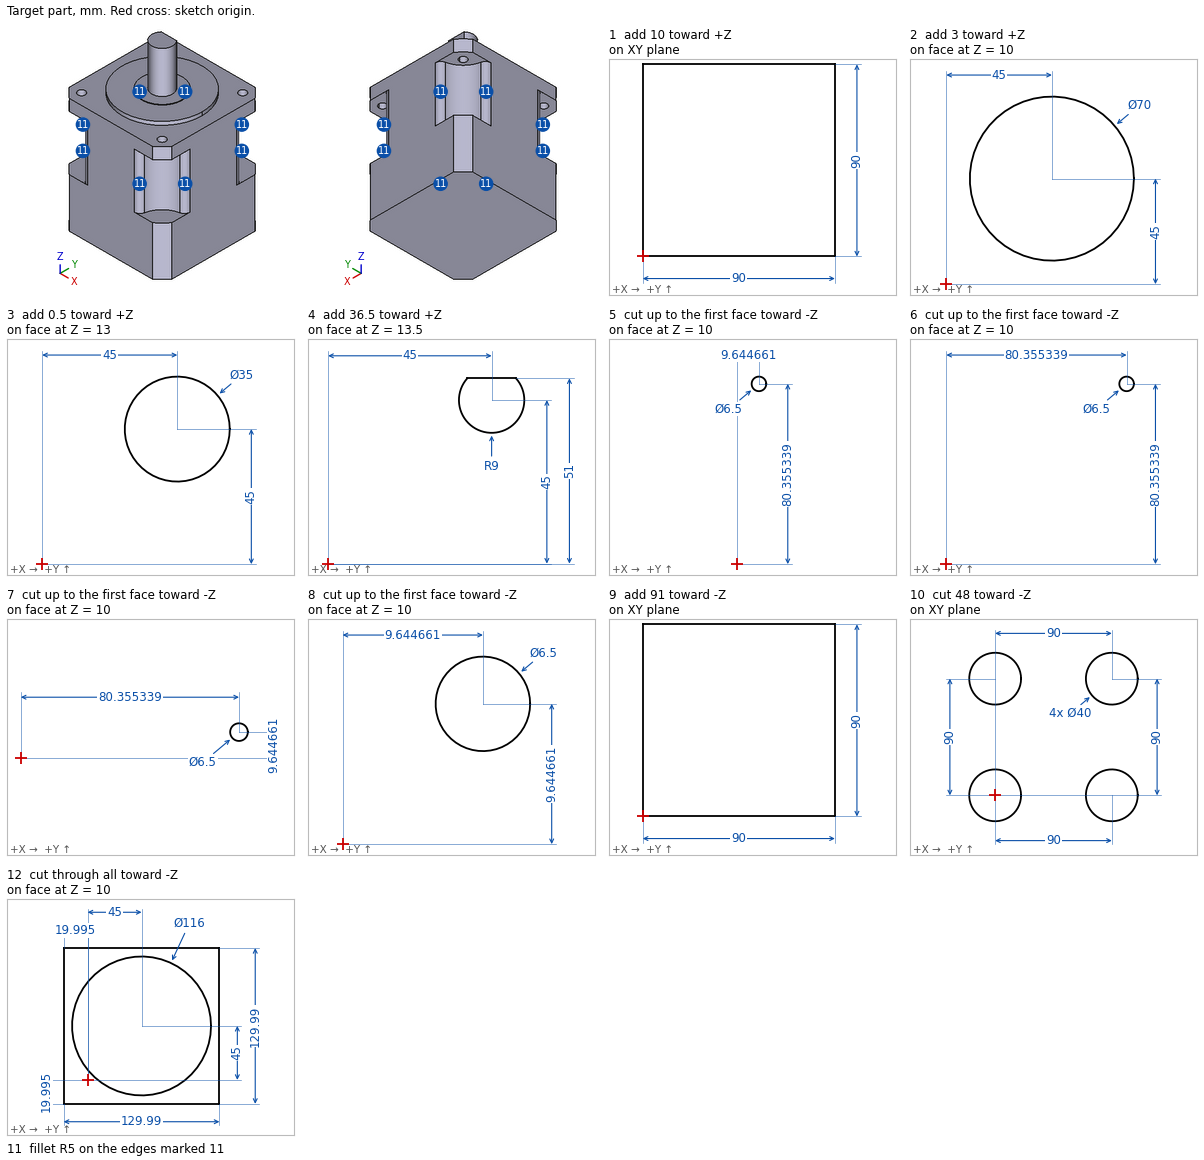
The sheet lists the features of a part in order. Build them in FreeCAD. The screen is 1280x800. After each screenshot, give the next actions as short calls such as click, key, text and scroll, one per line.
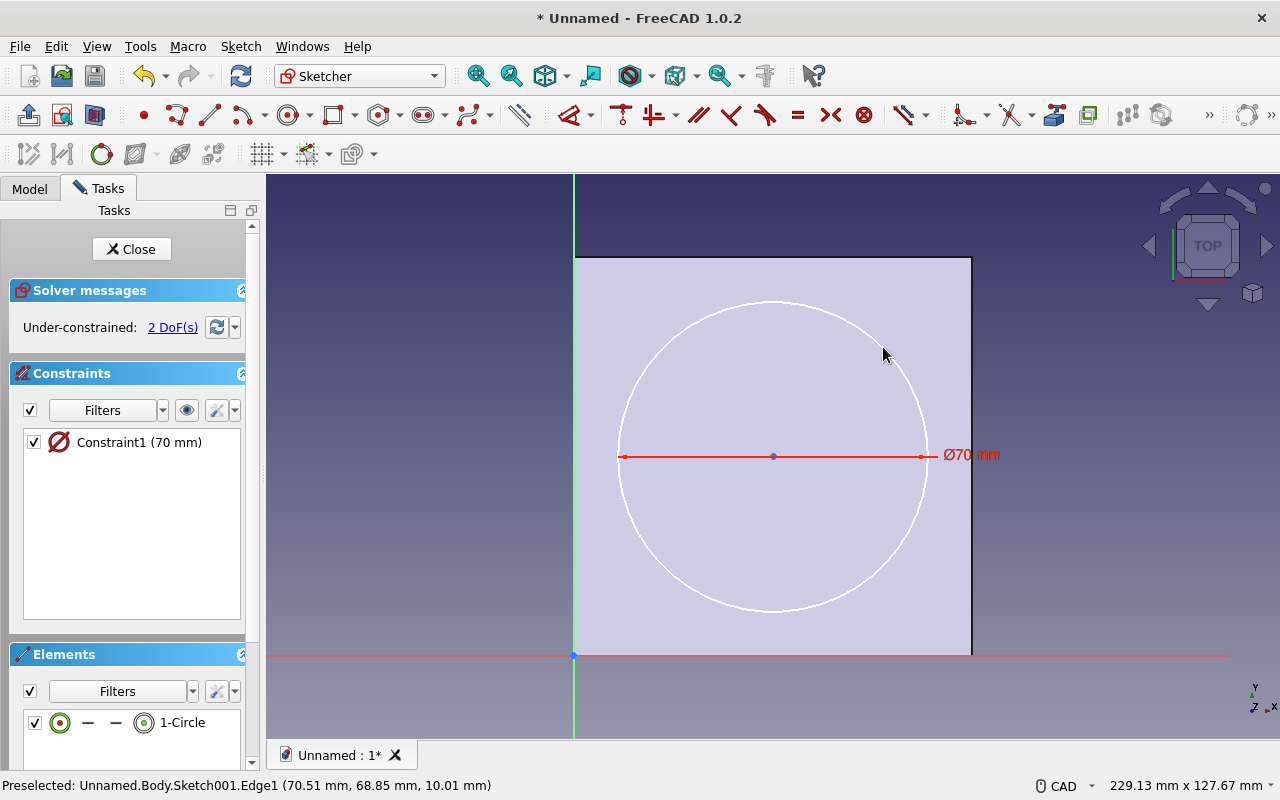
click(773, 457)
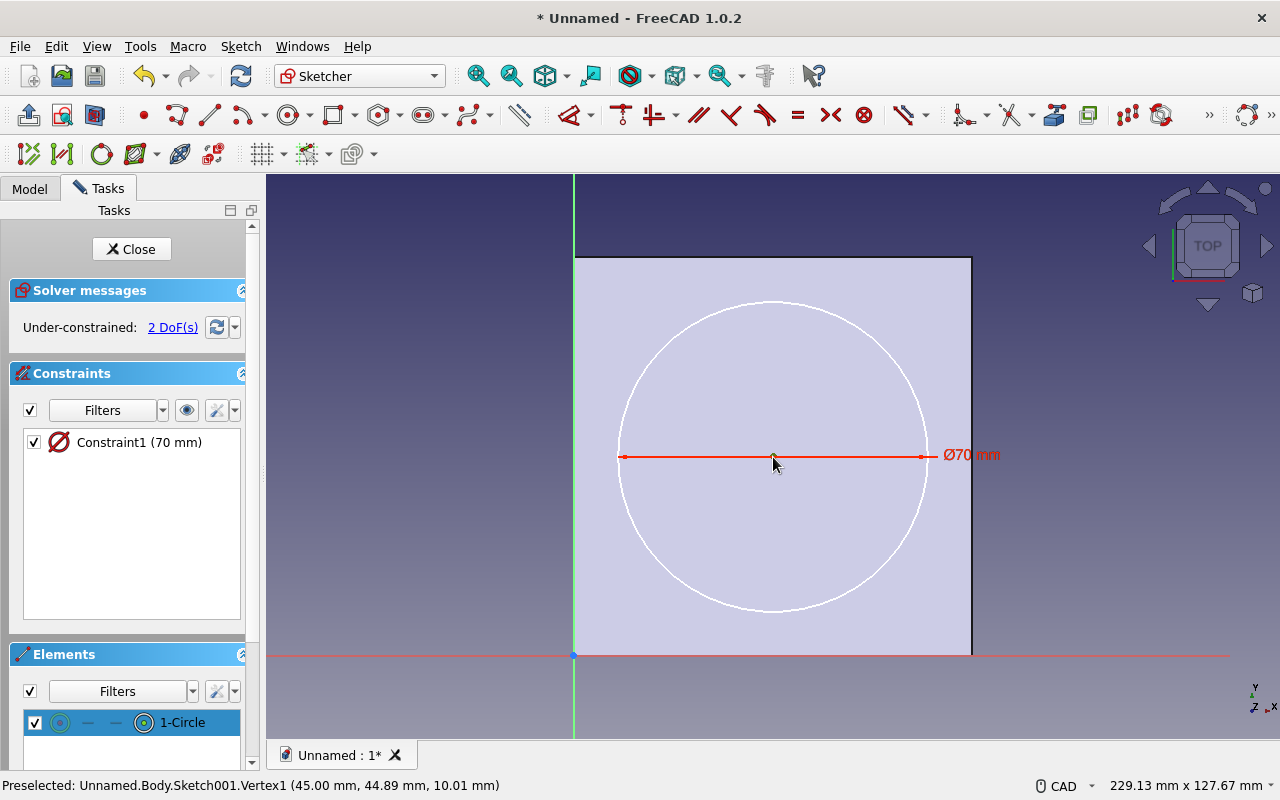
key(l)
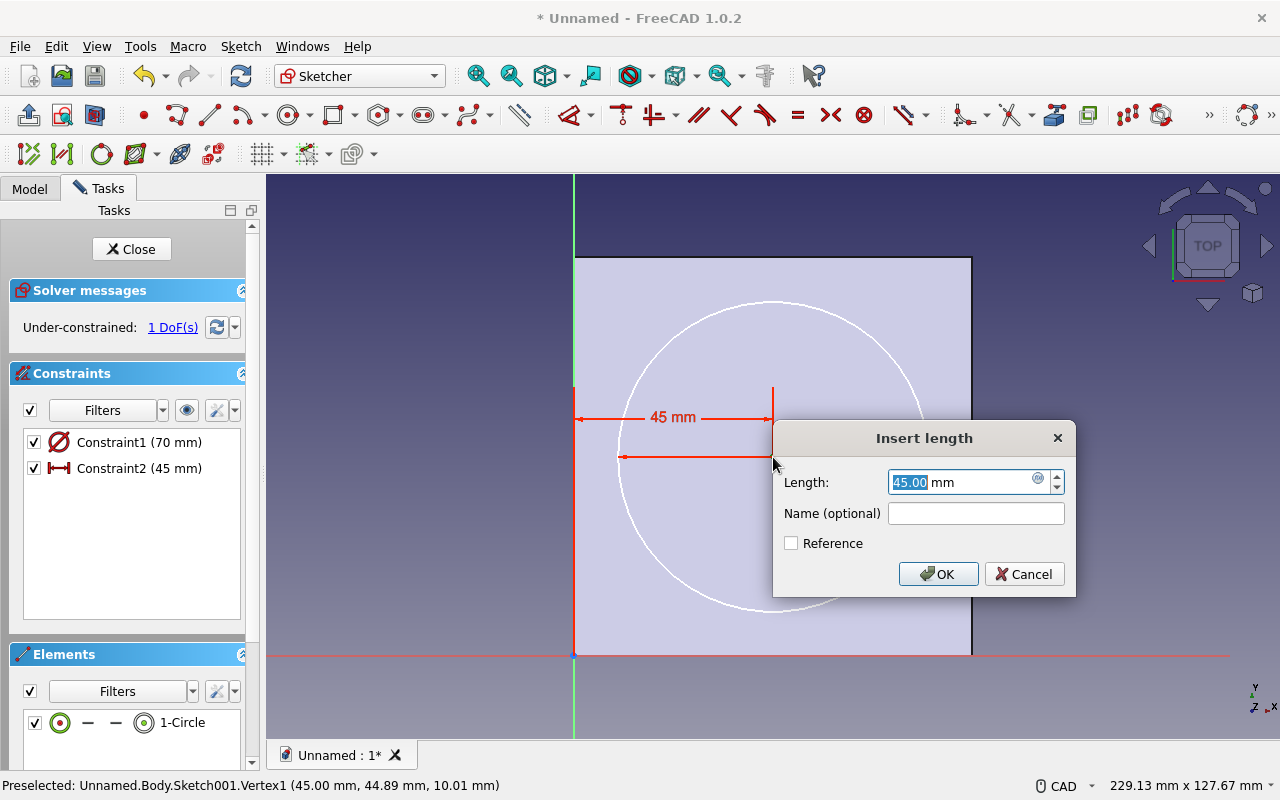
text(45)
key(Return)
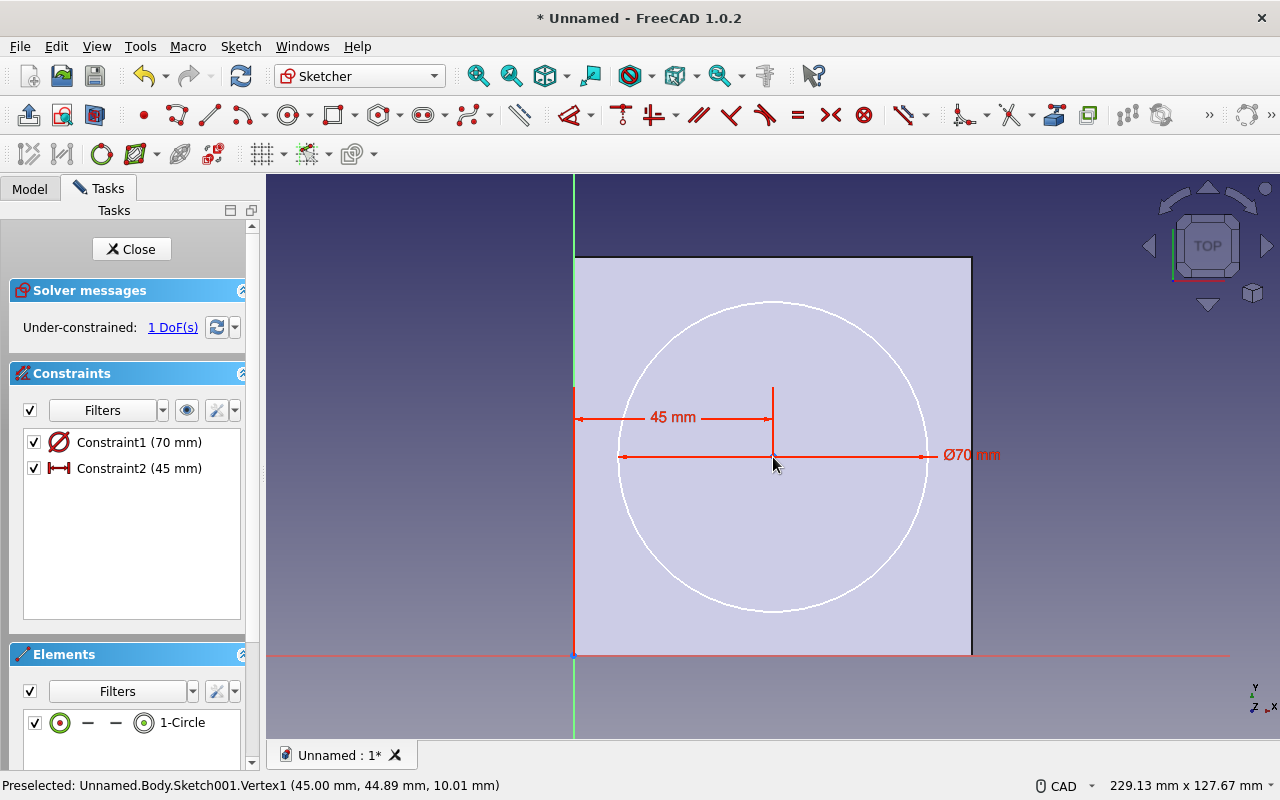
click(773, 457)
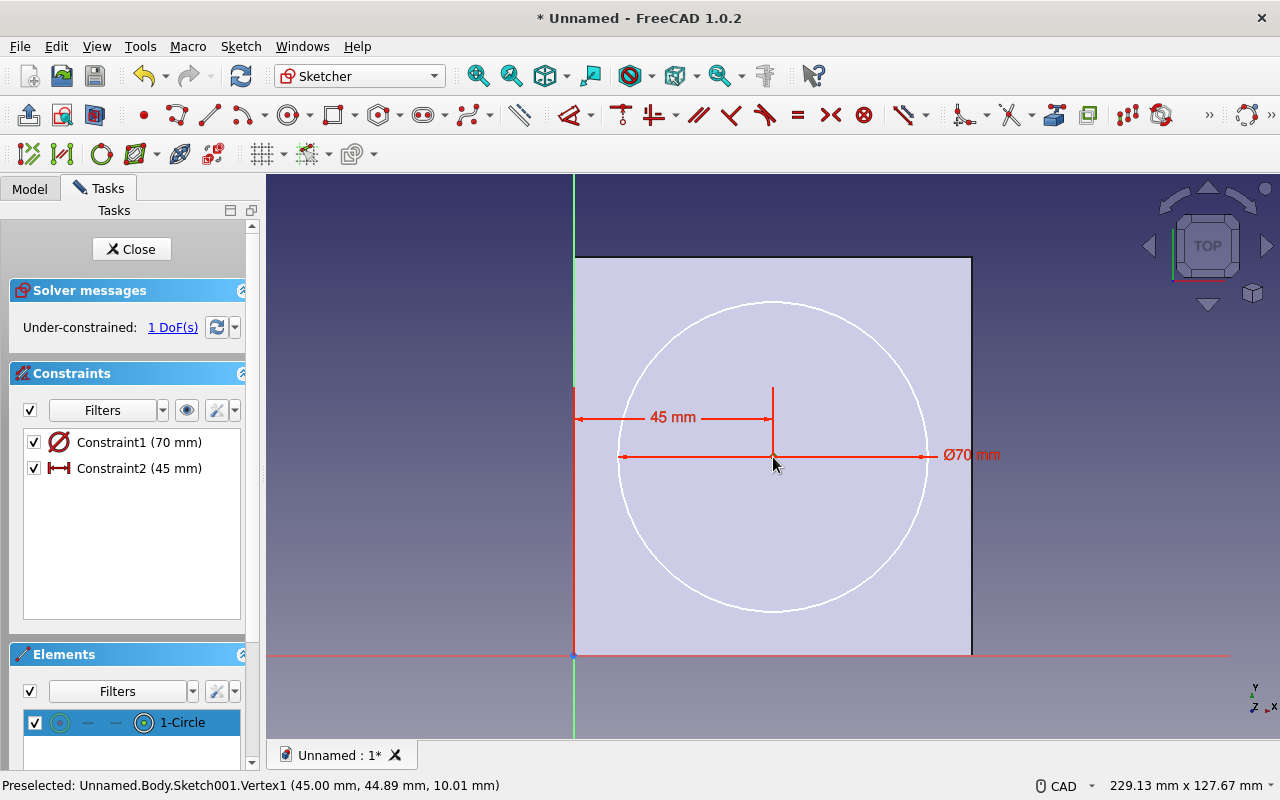
key(i)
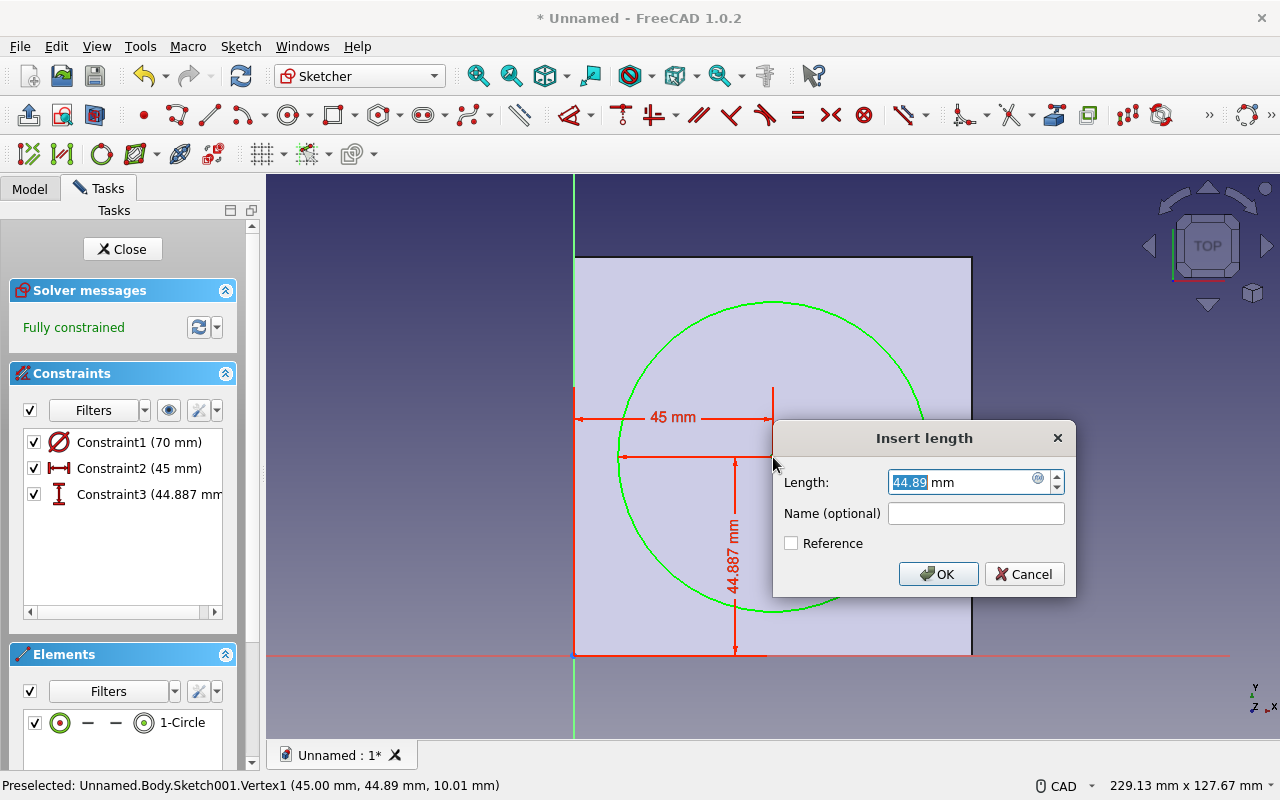
text(45)
key(Return)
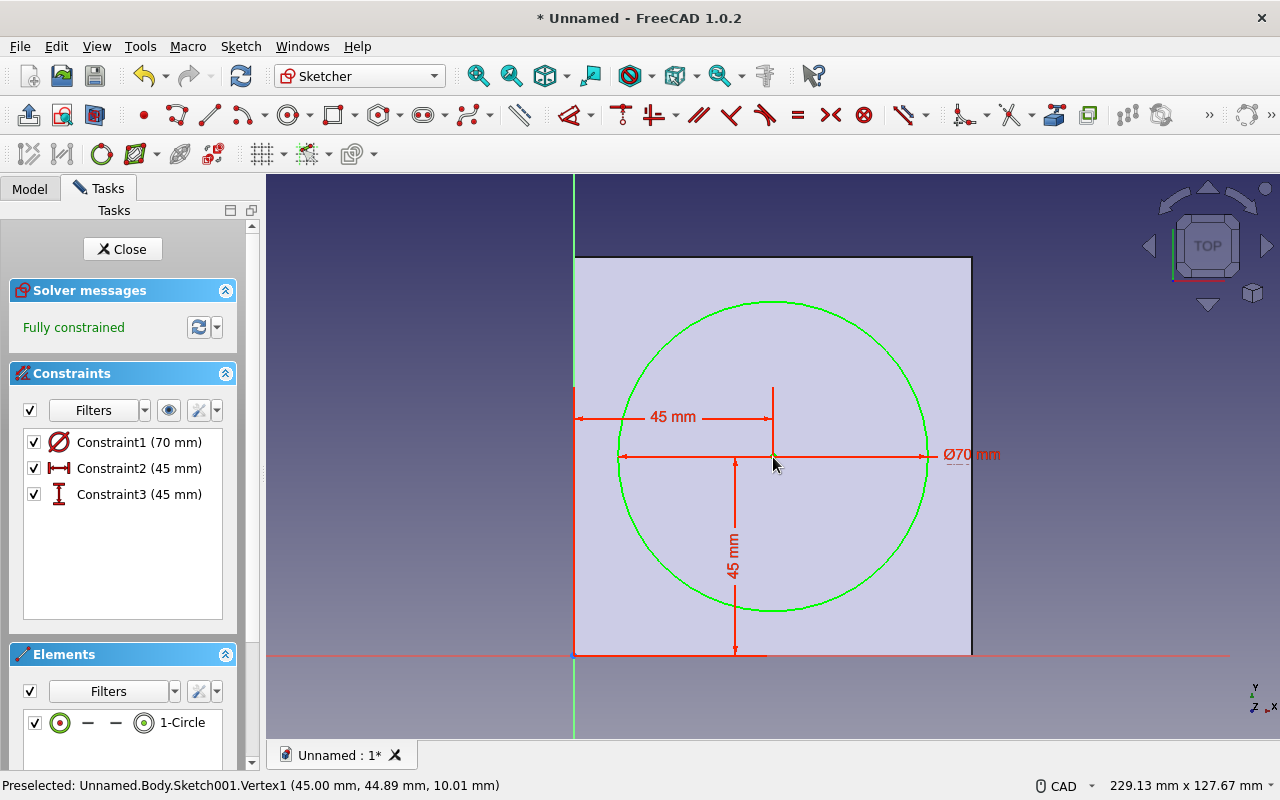
click(123, 249)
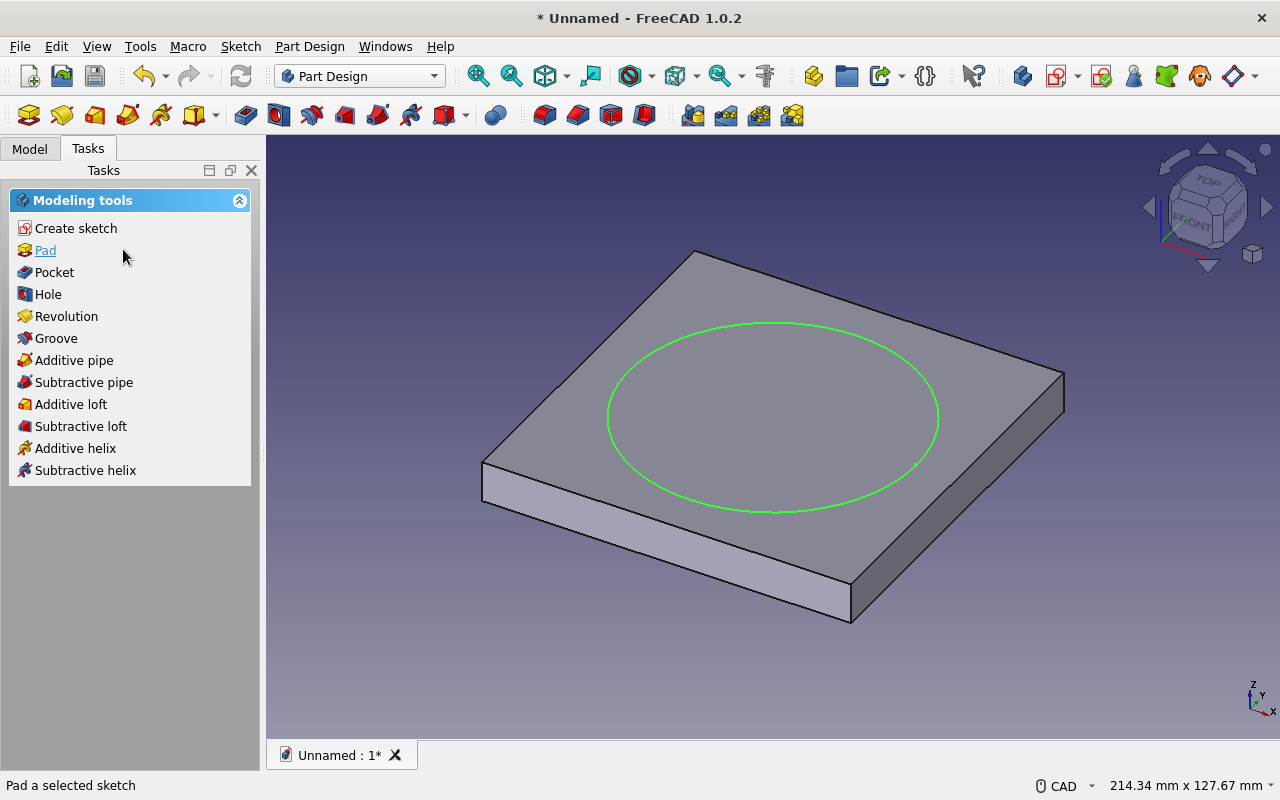
click(29, 116)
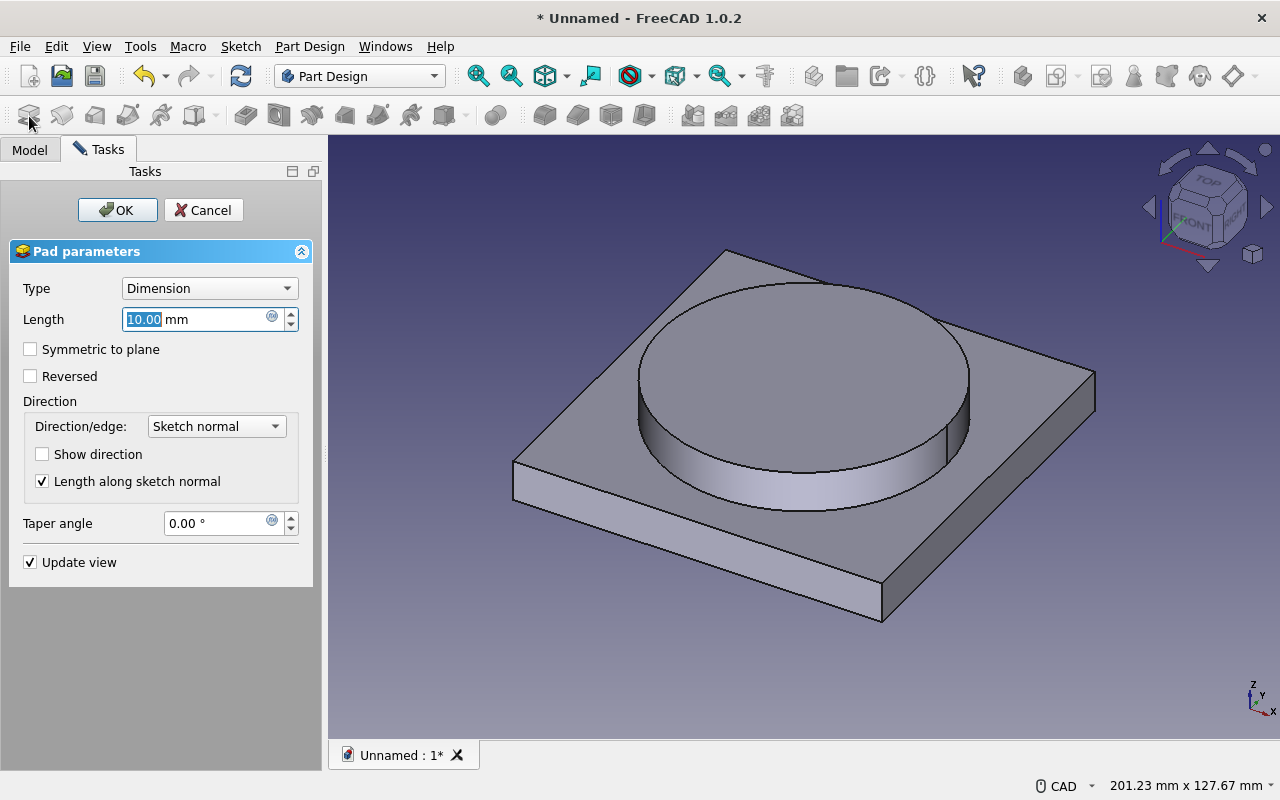
text(3)
key(Tab)